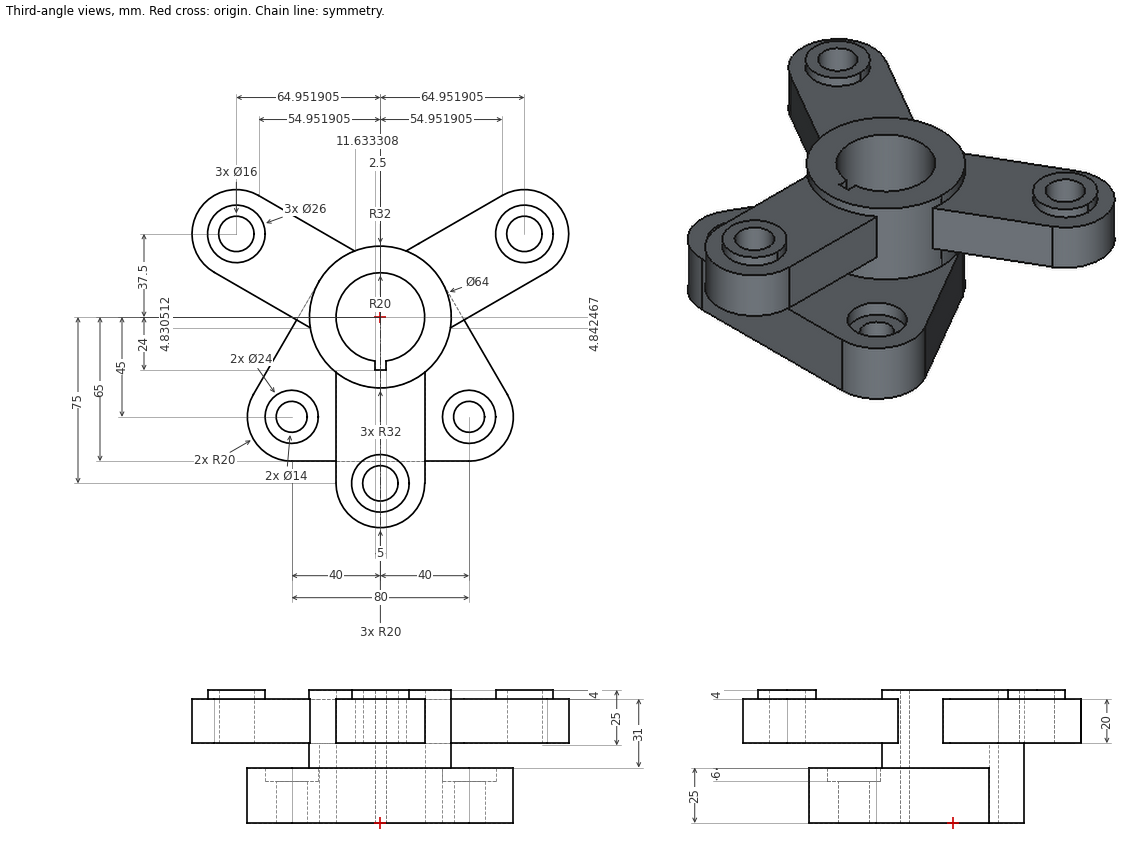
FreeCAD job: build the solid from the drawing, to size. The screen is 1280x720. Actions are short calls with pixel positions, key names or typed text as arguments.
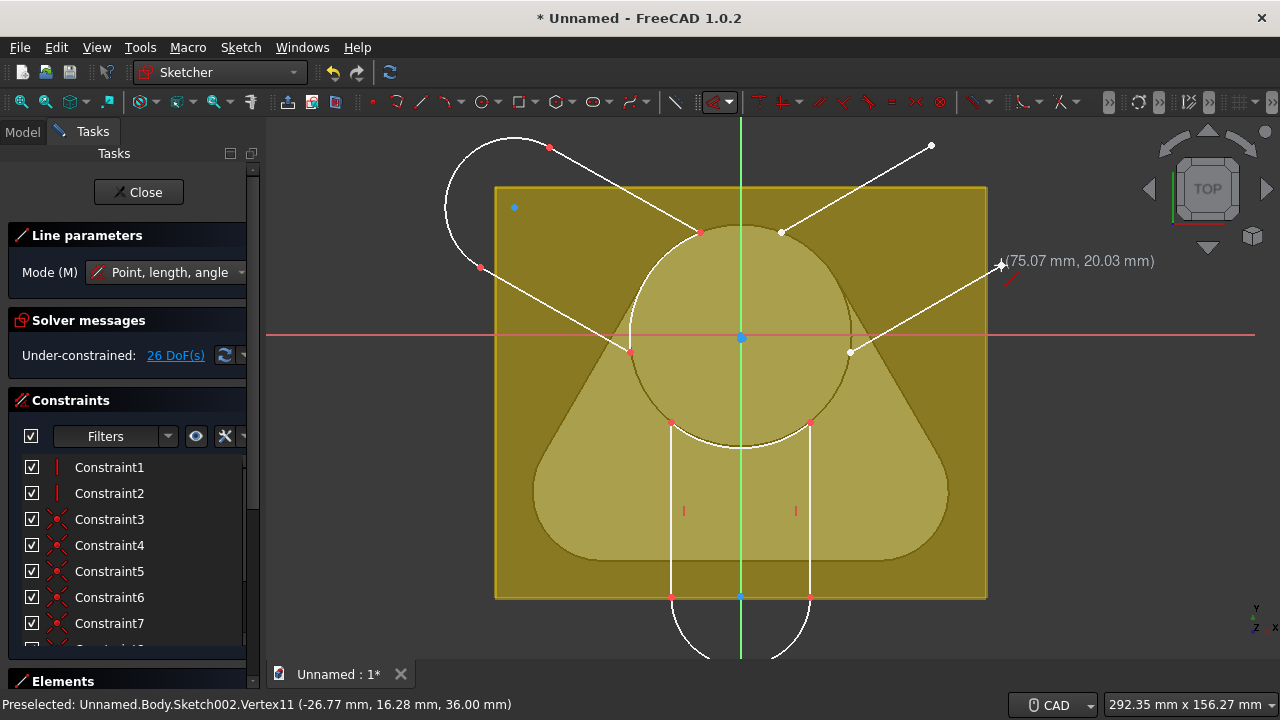
key(g)
key(3)
key(a)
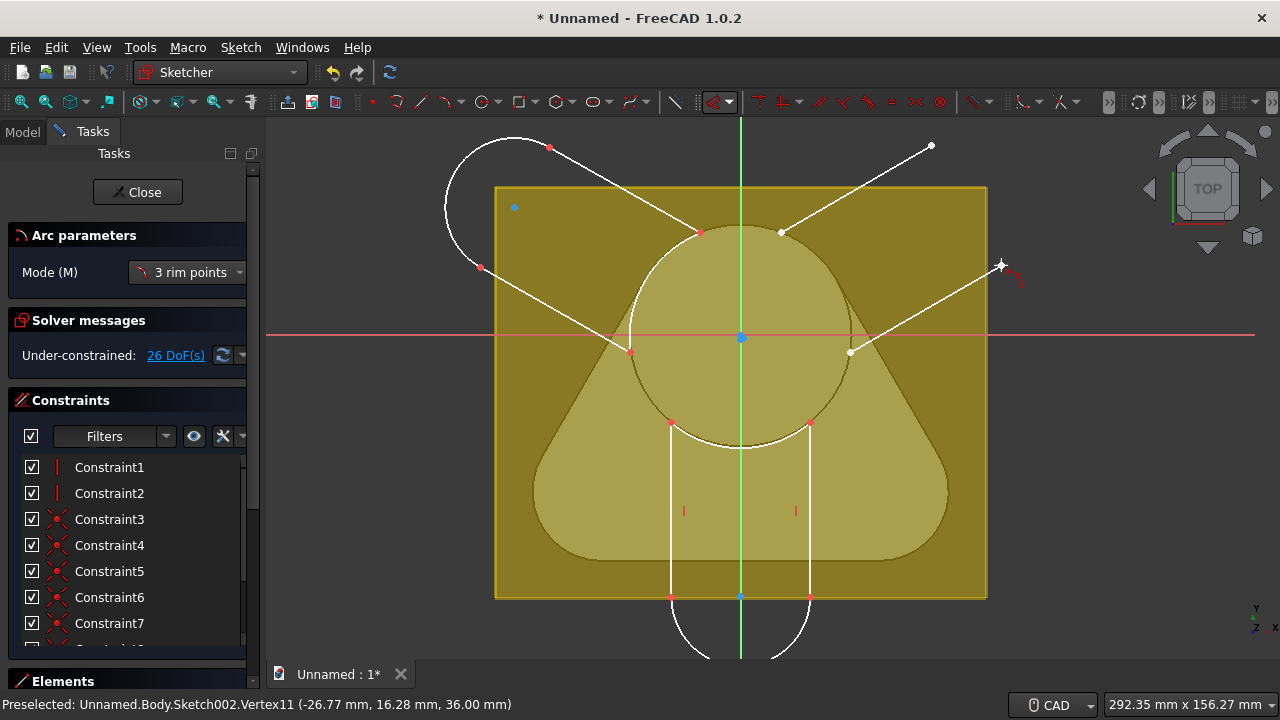
click(781, 233)
click(850, 353)
click(837, 280)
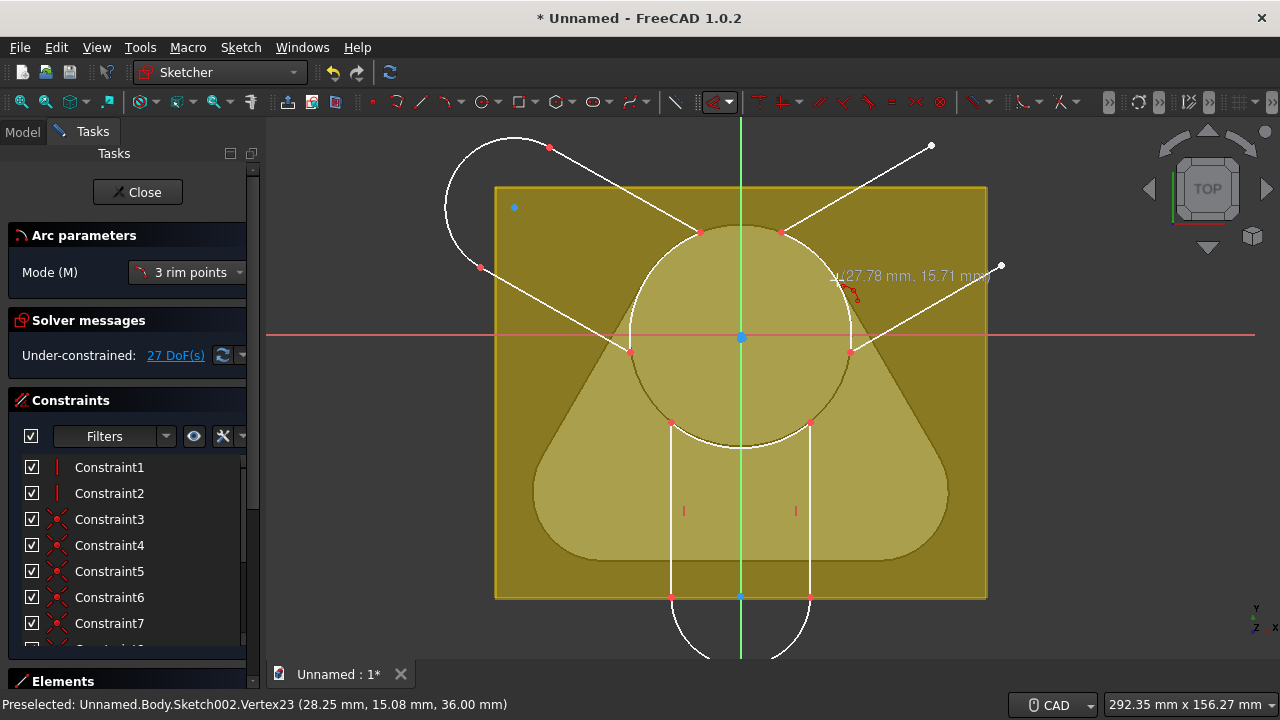
click(1001, 266)
click(931, 146)
click(1026, 171)
key(Escape)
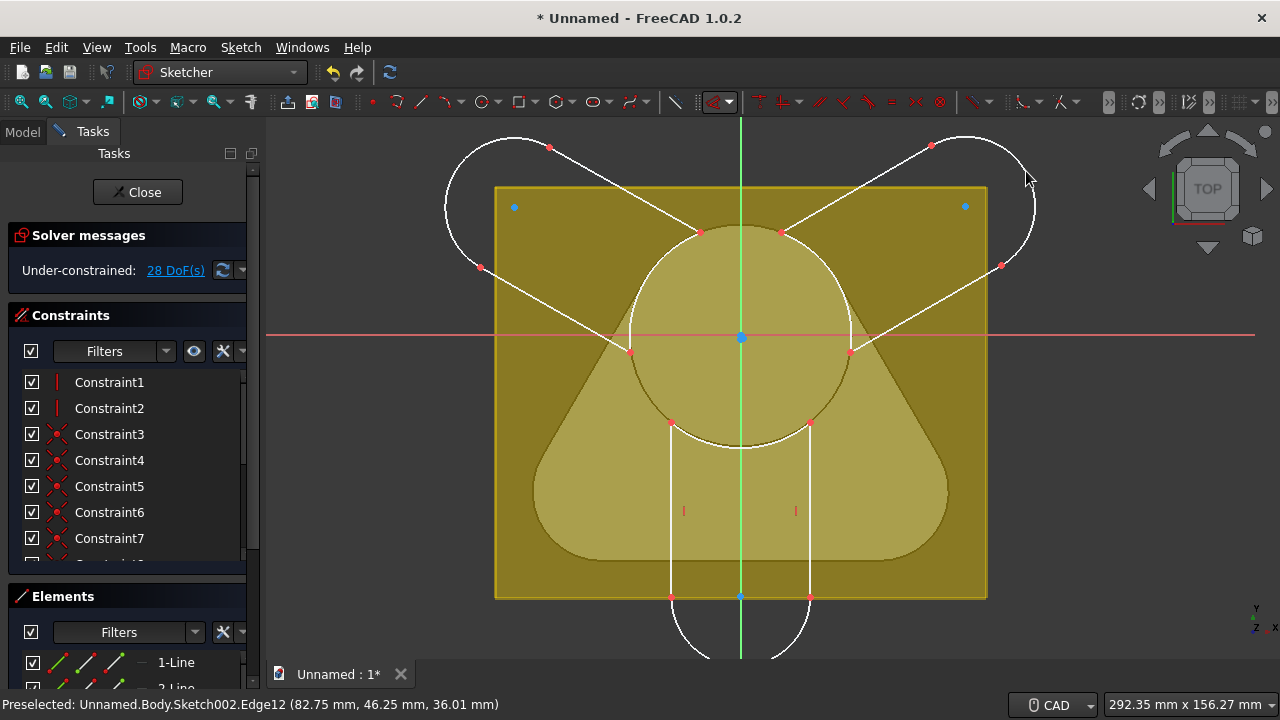
click(671, 475)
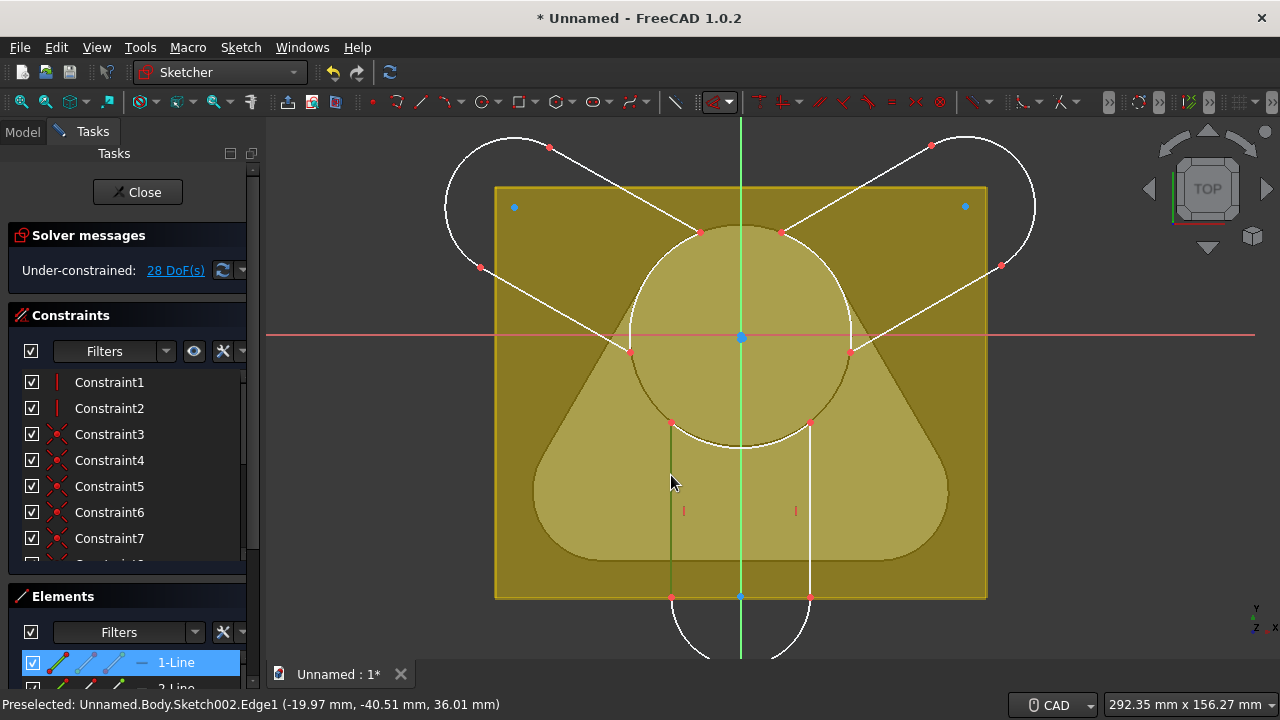
scroll(631, 353, down, 2)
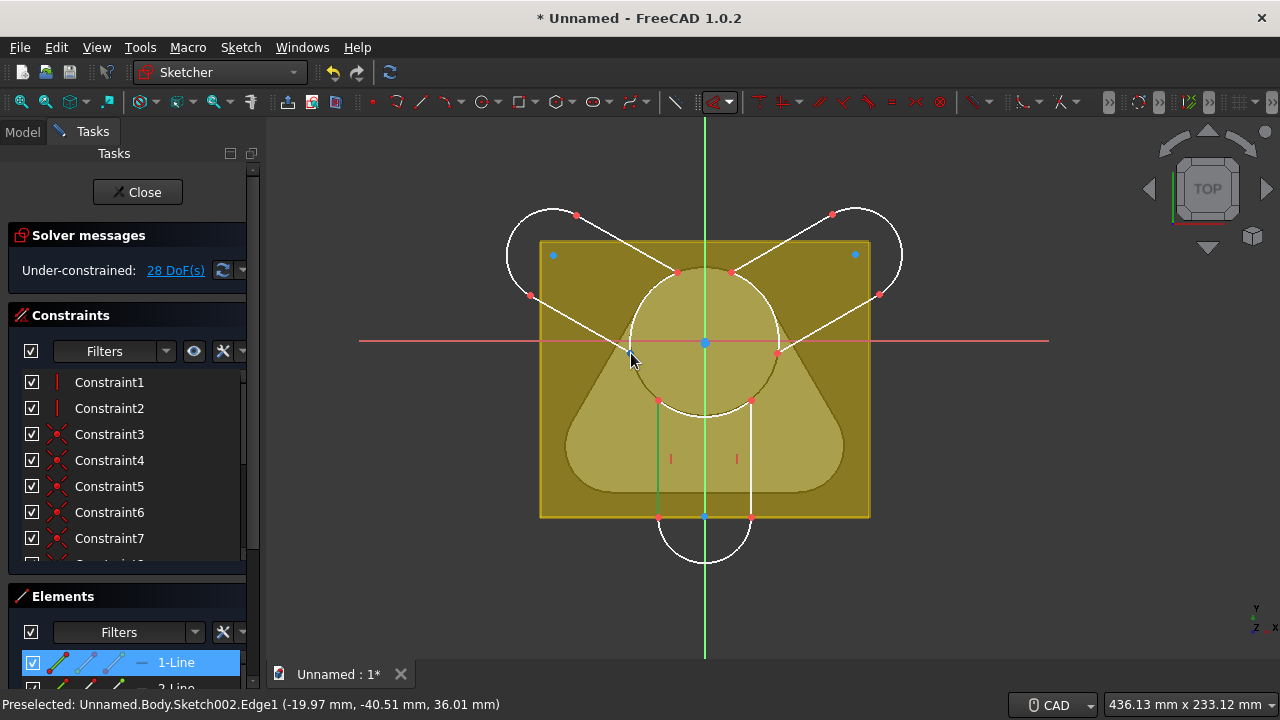
click(677, 554)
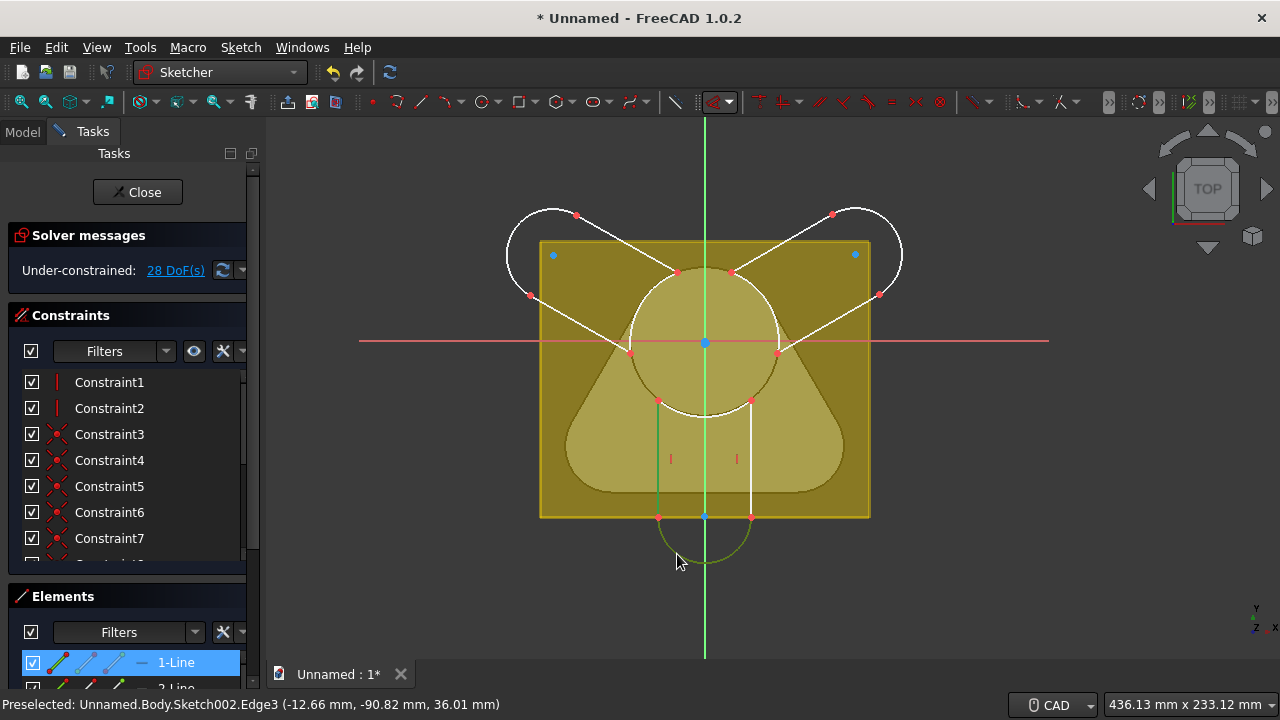
click(868, 102)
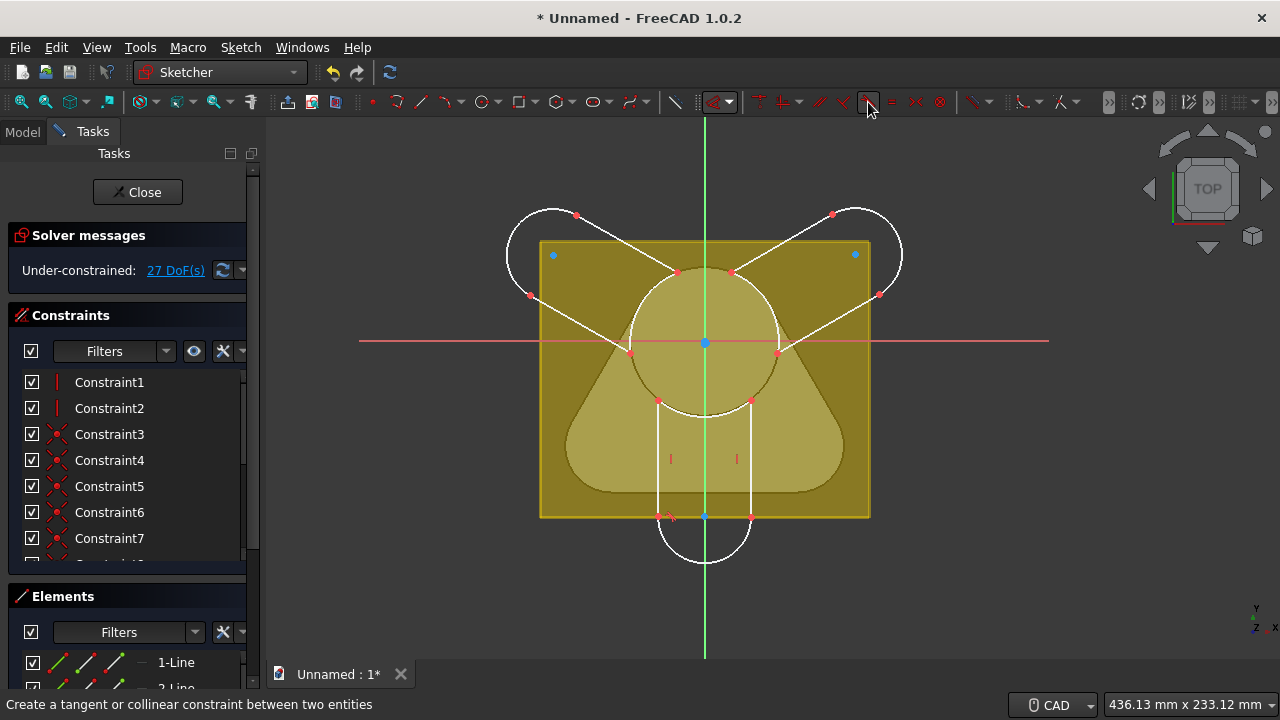
click(751, 482)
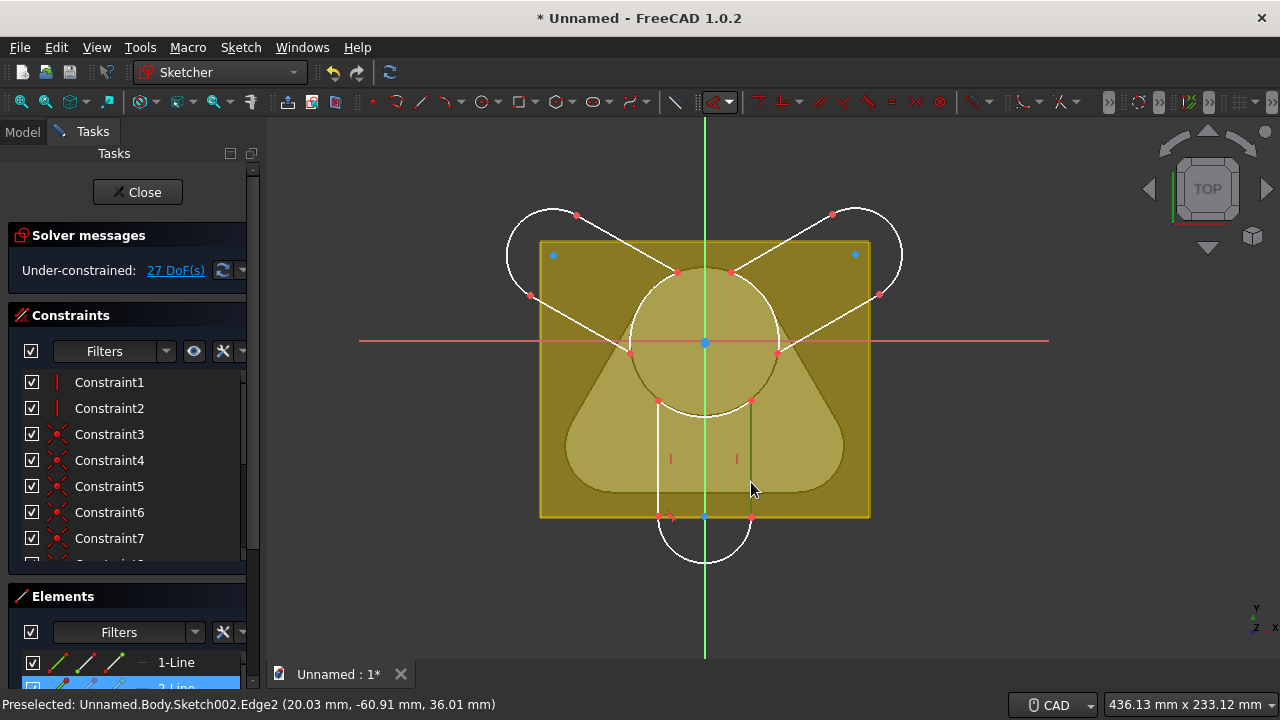
click(677, 554)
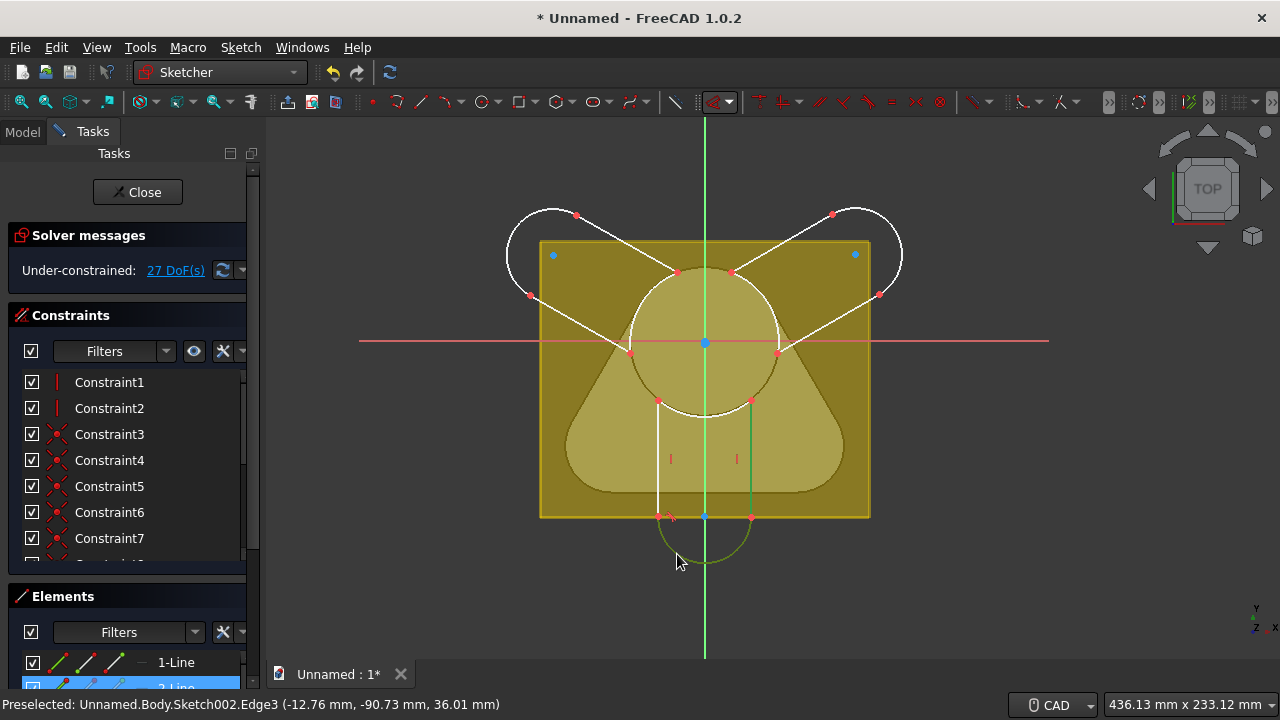
key(t)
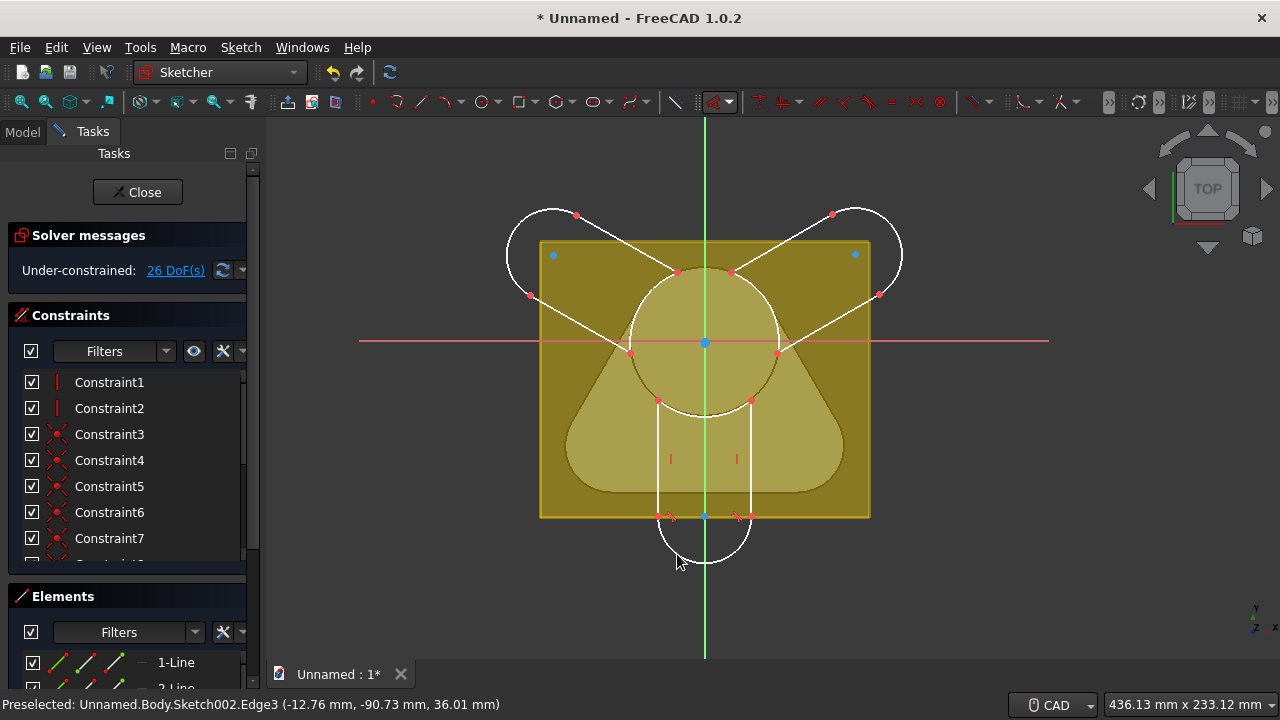
click(647, 255)